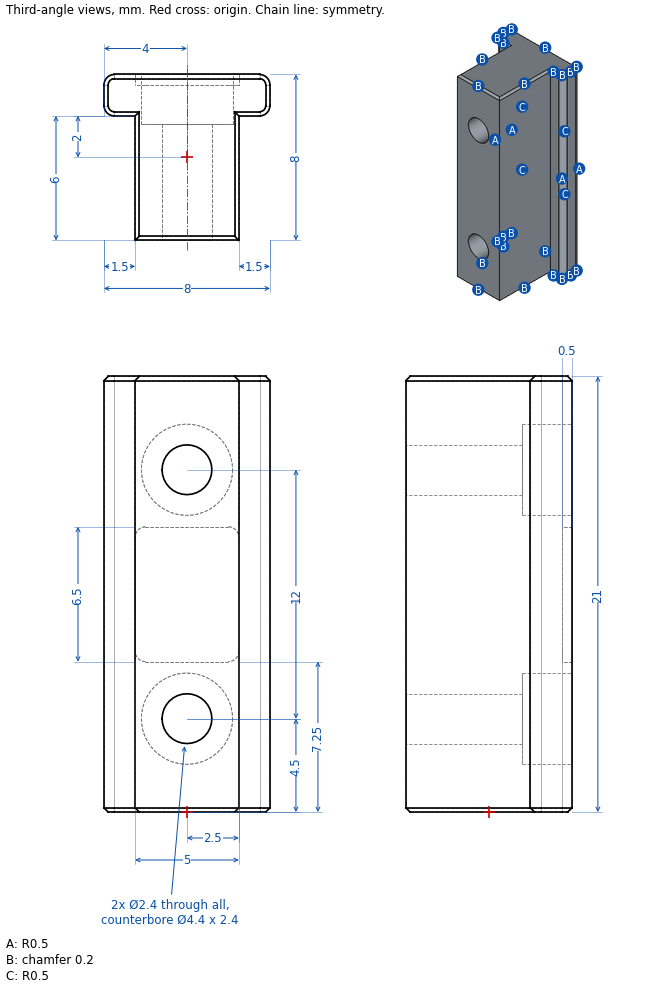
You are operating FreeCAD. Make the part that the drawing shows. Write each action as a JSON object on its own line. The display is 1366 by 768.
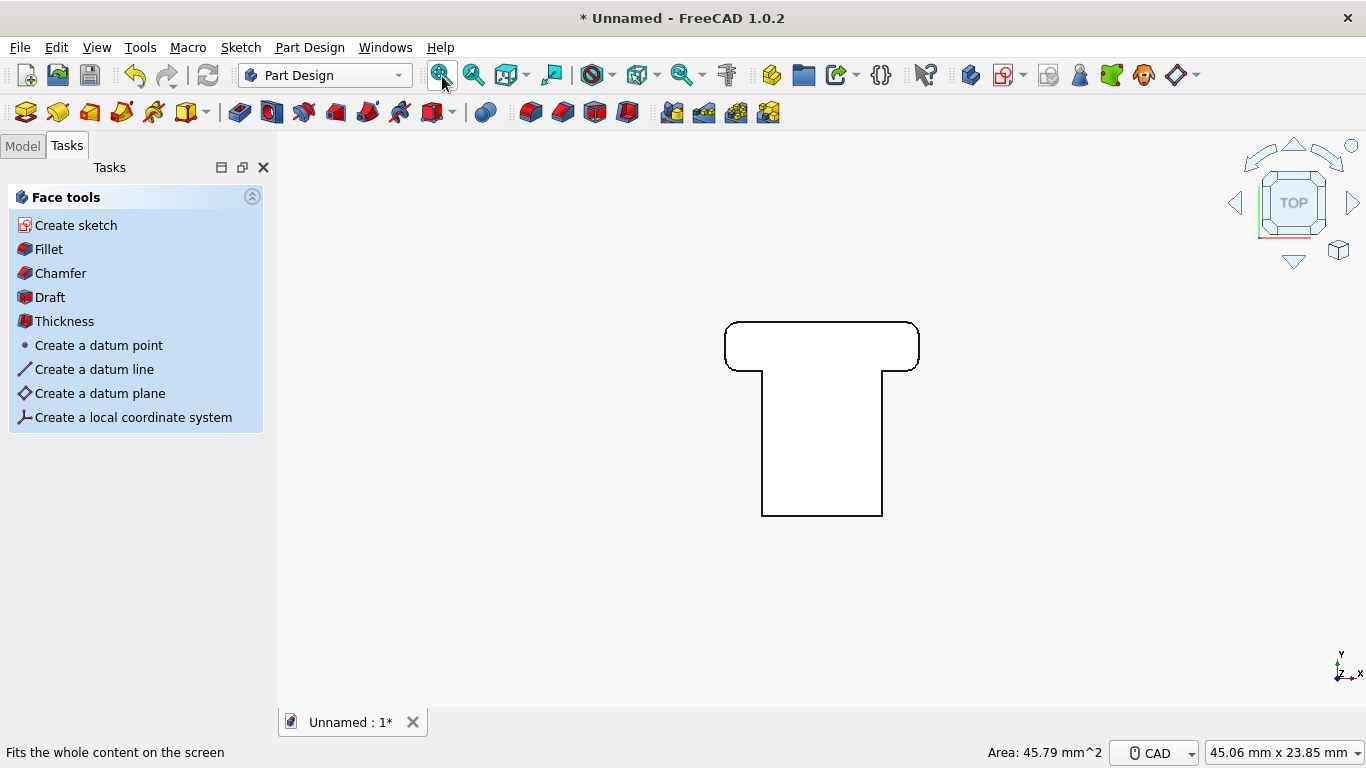
{"action": "key", "text": "1"}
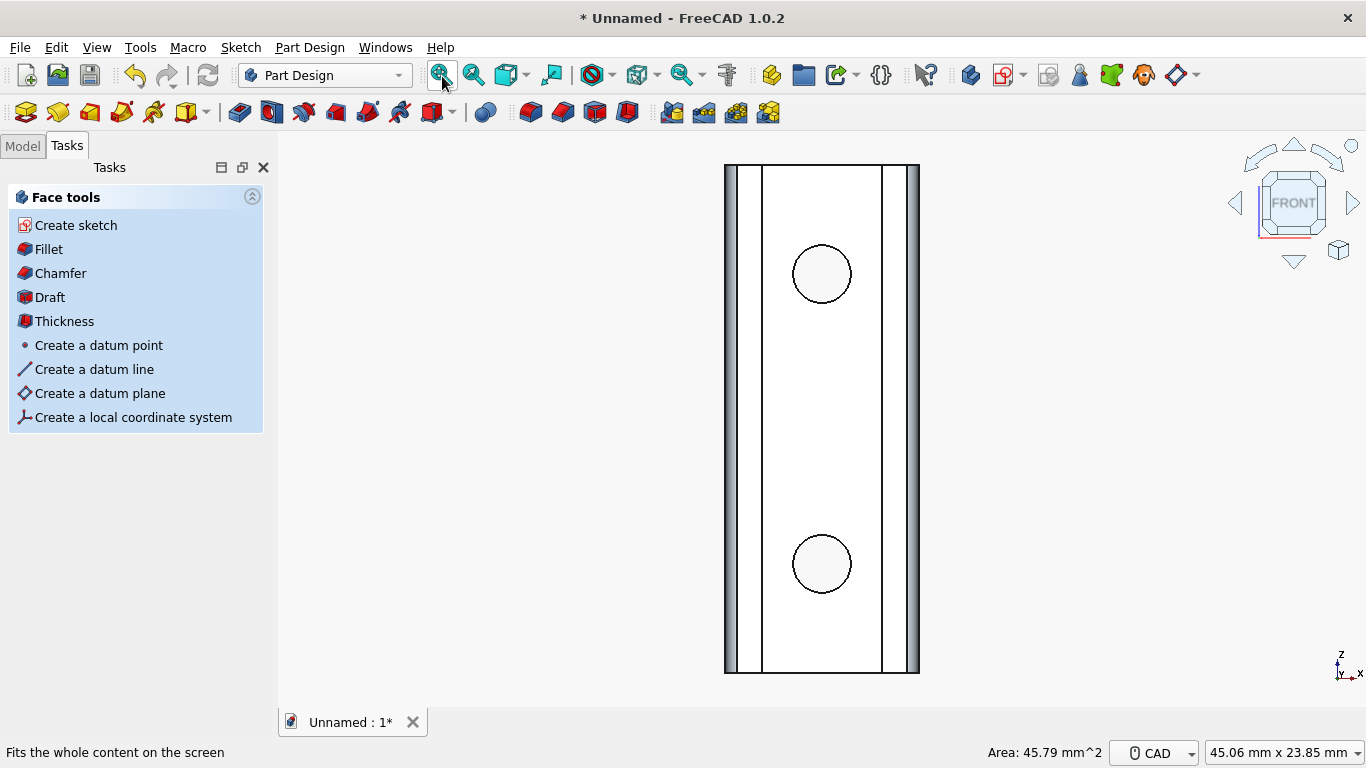
{"action": "key", "text": "3"}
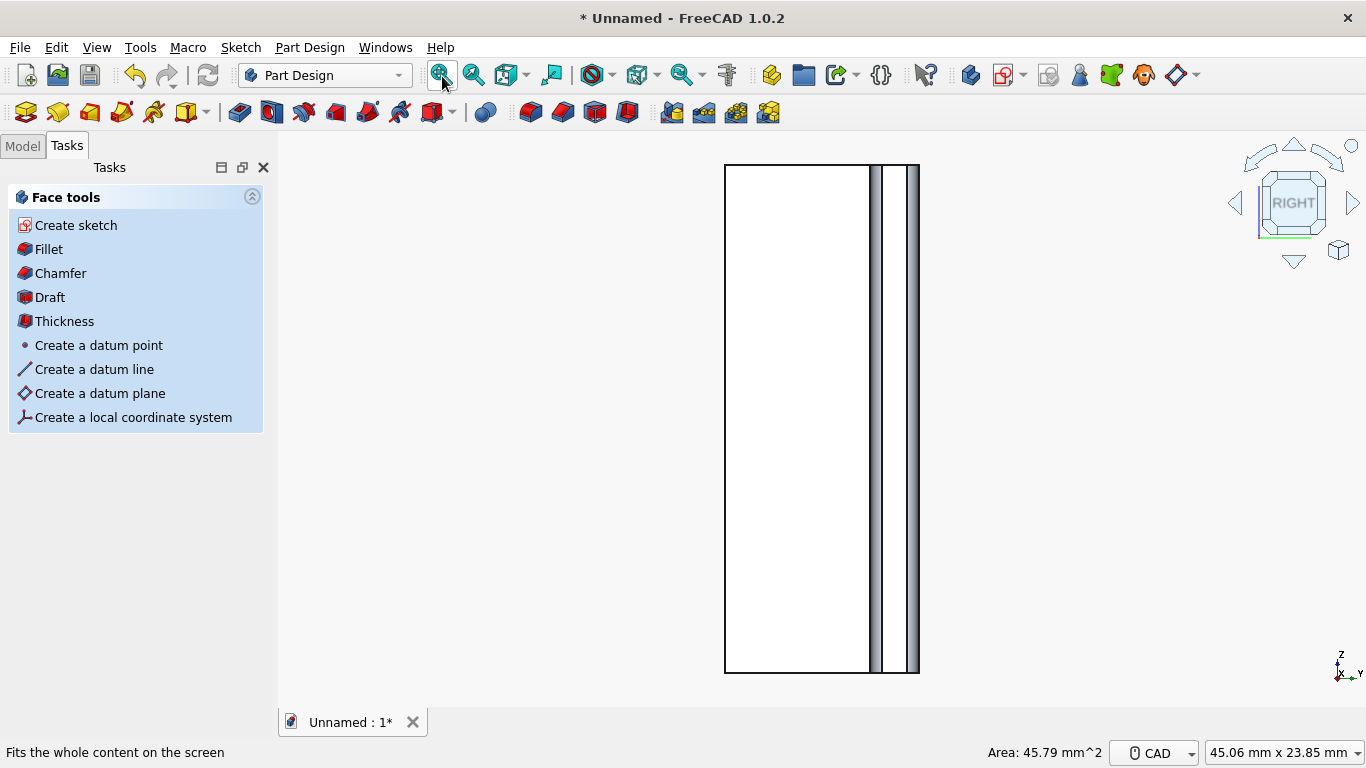
{"action": "key", "text": "5"}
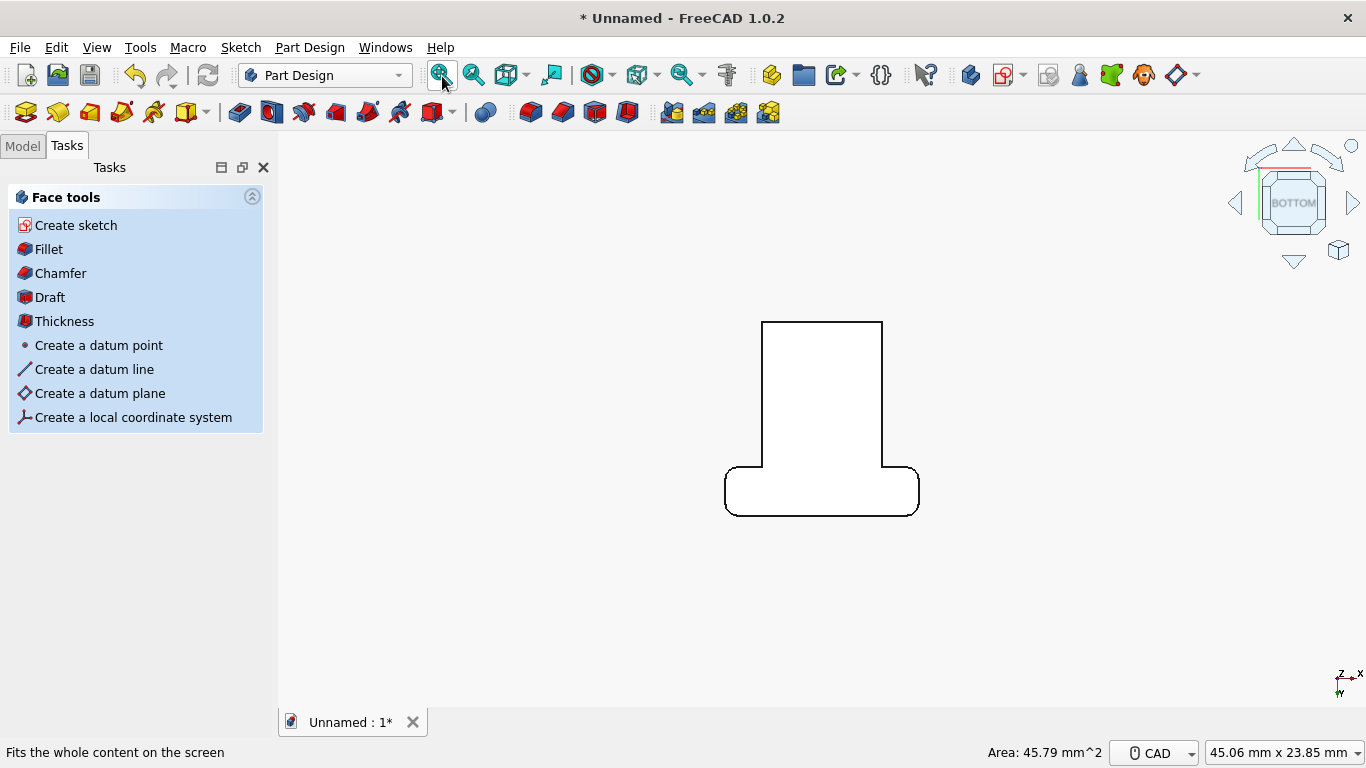
{"action": "left_click", "coordinate": [442, 76]}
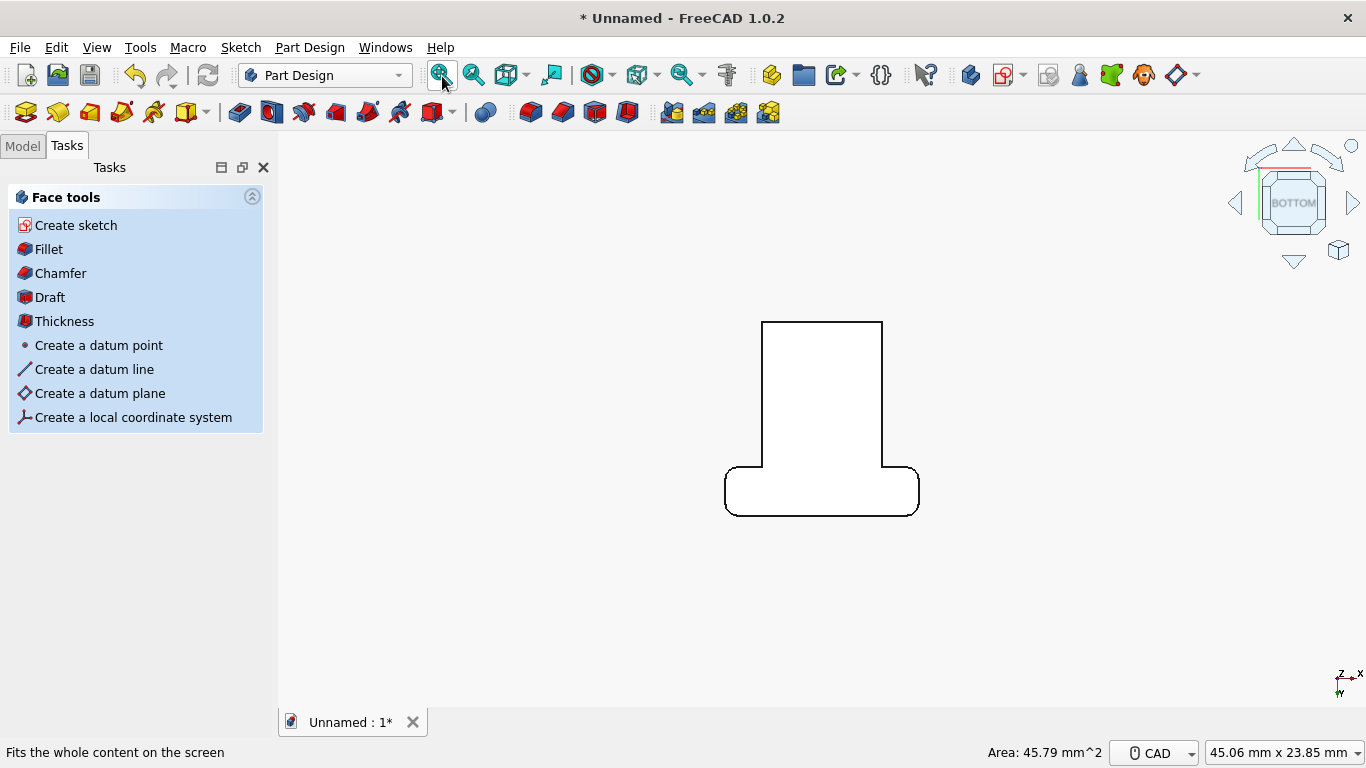
{"action": "left_click", "coordinate": [822, 446], "text": "ctrl"}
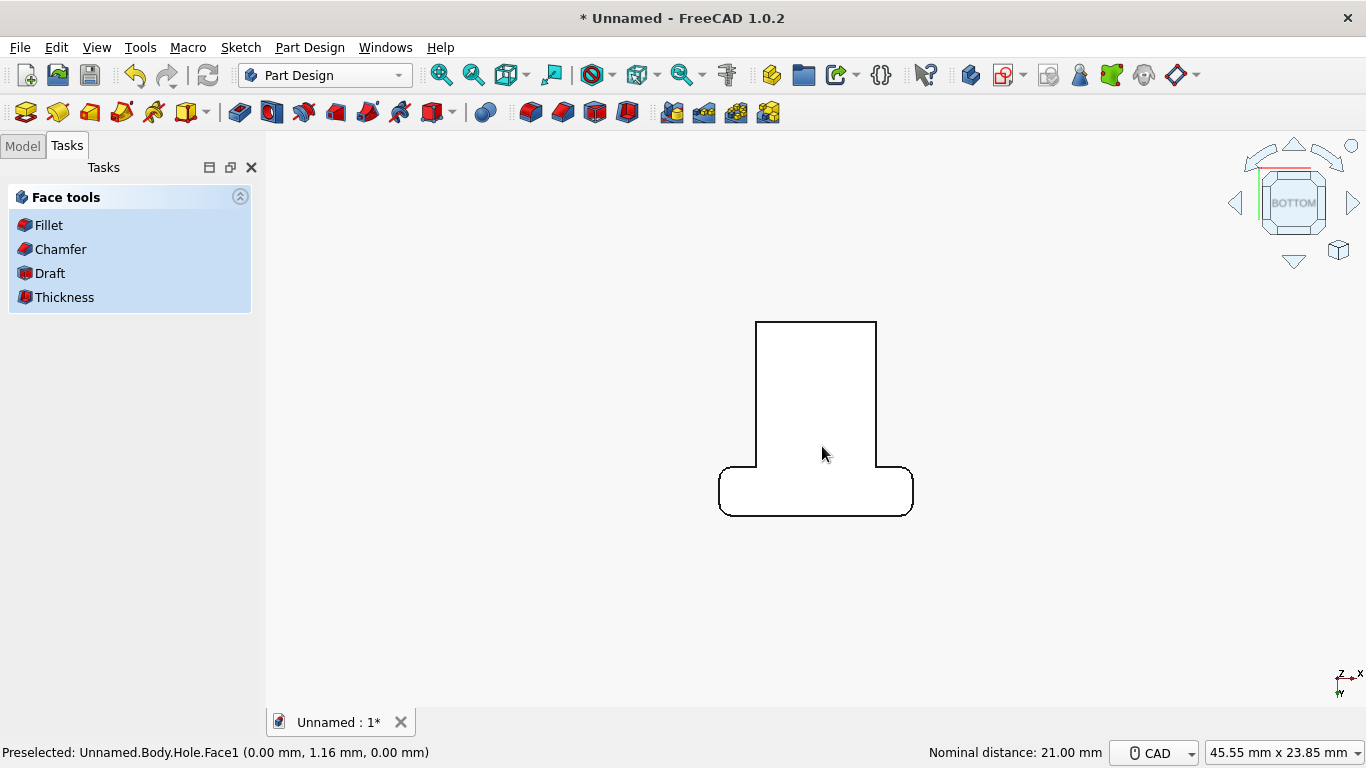
{"action": "left_click", "coordinate": [564, 112]}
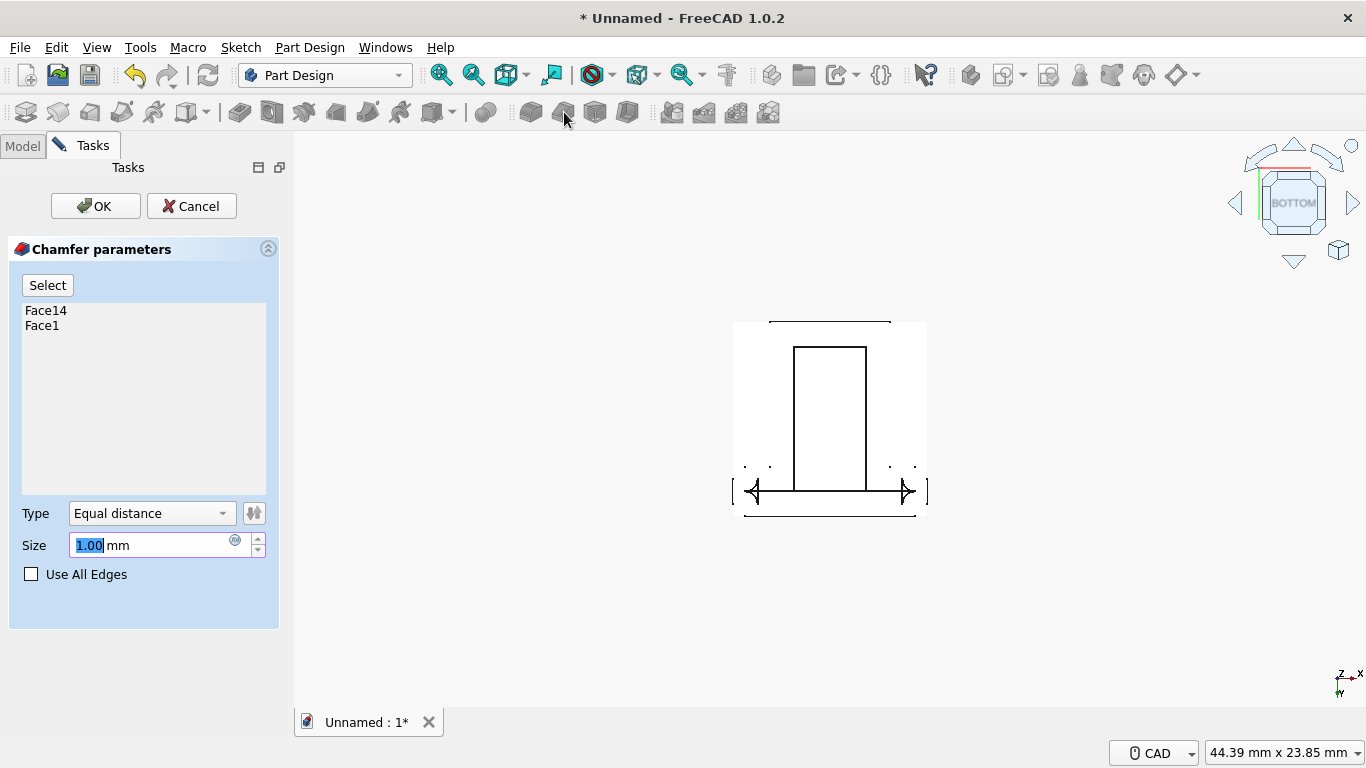
{"action": "type", "text": "0.2"}
{"action": "key", "text": "Tab"}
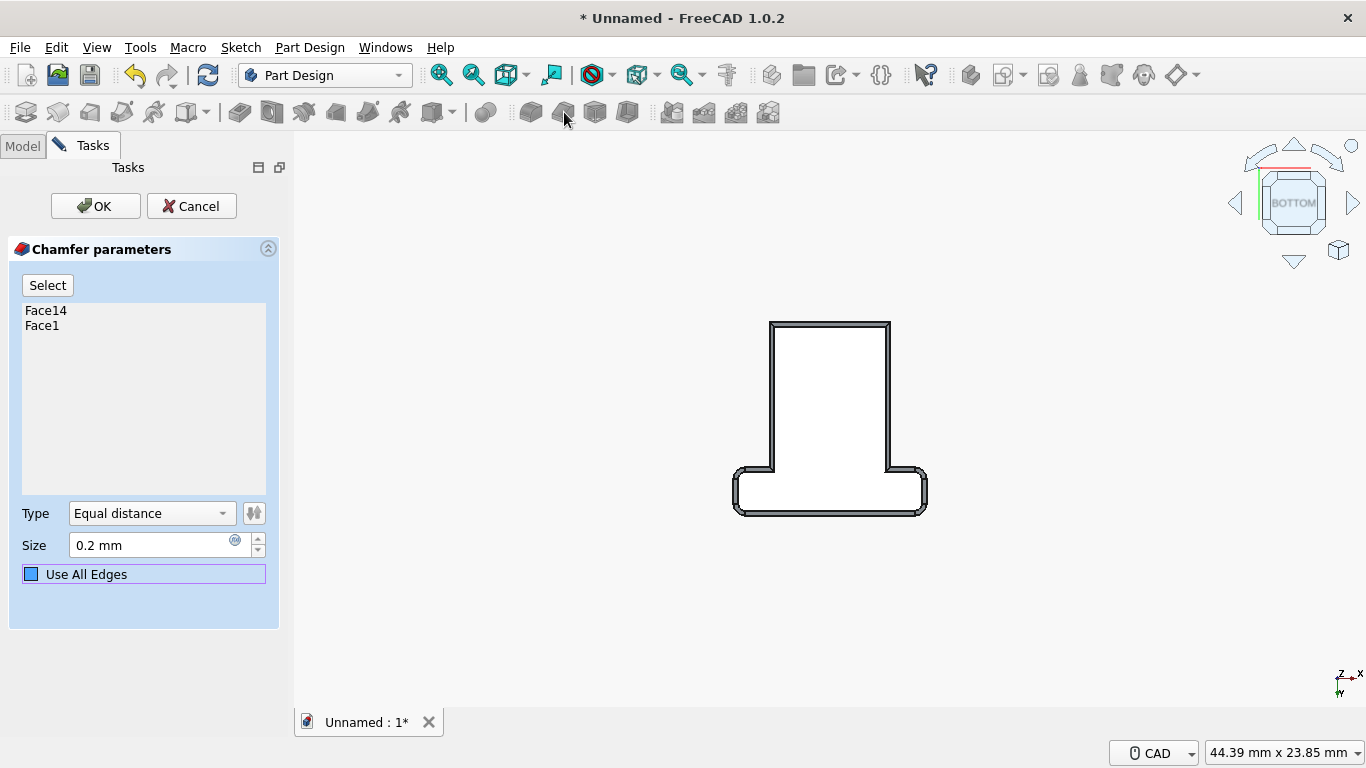
{"action": "left_click", "coordinate": [96, 206]}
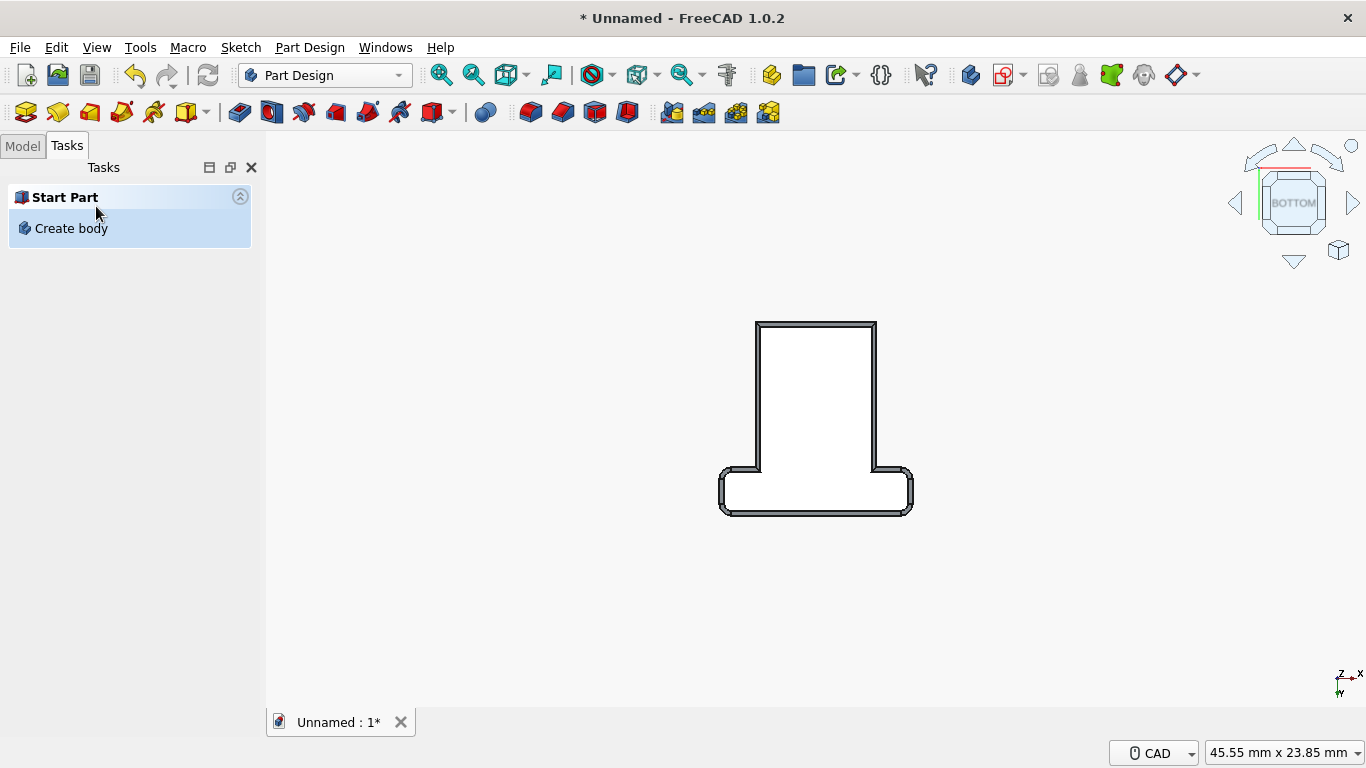
{"action": "left_click", "coordinate": [442, 76]}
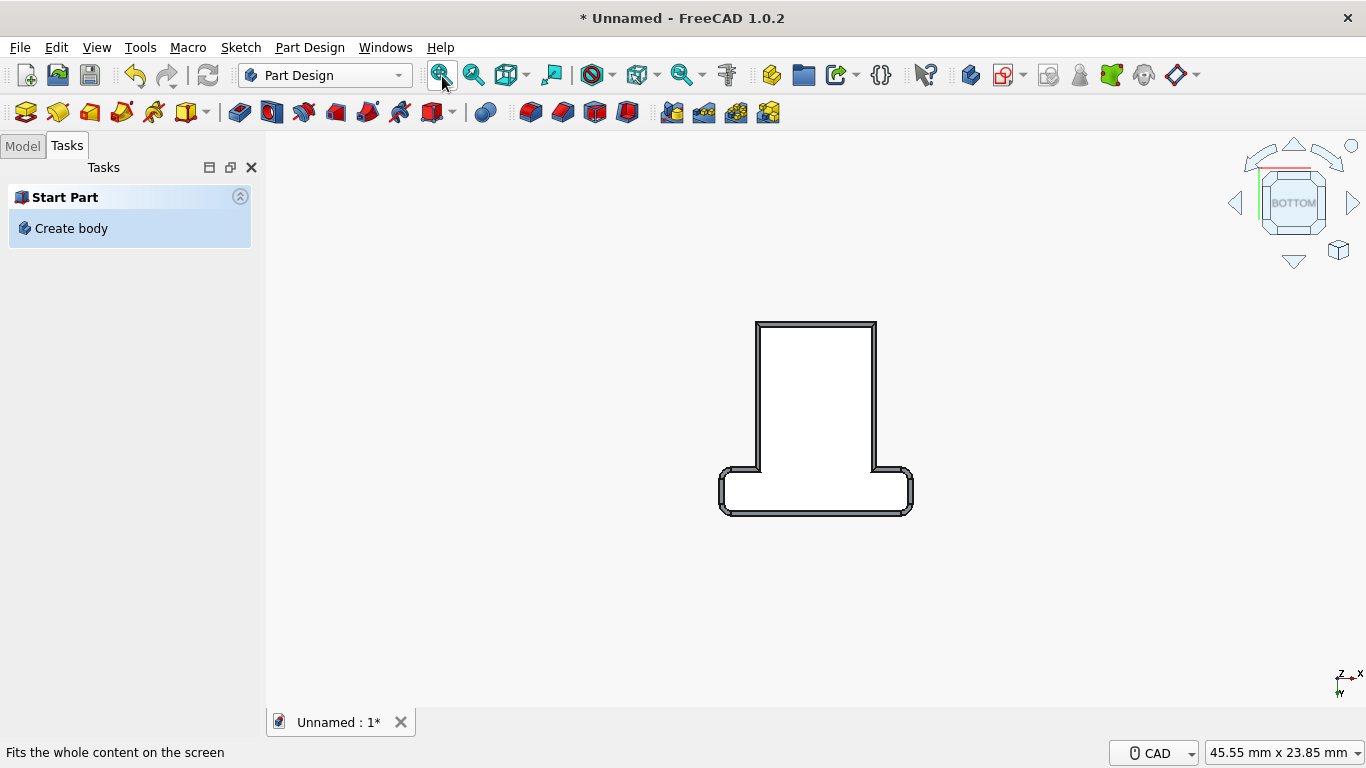
{"action": "key", "text": "4"}